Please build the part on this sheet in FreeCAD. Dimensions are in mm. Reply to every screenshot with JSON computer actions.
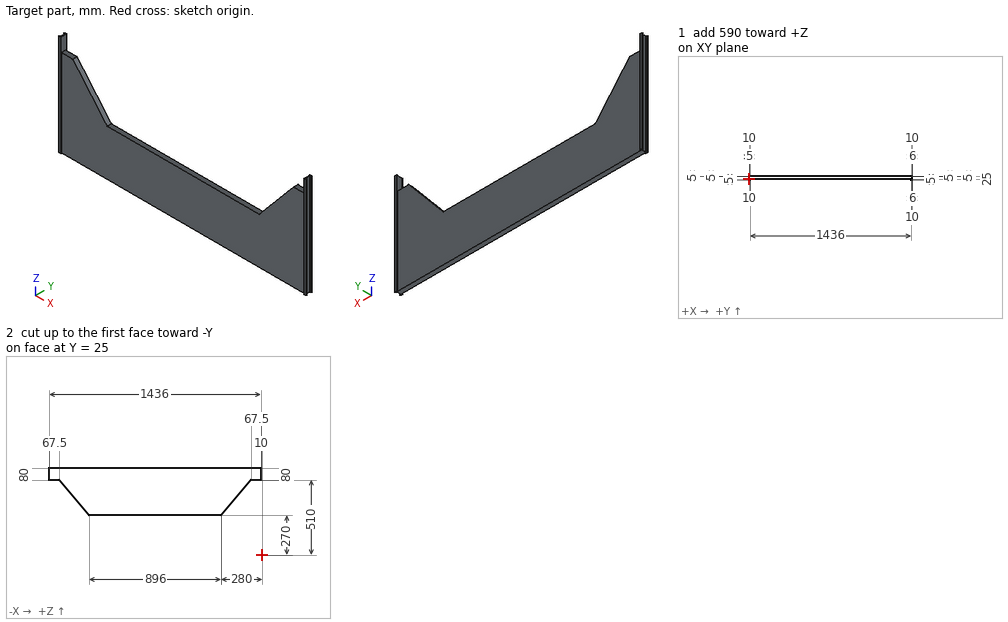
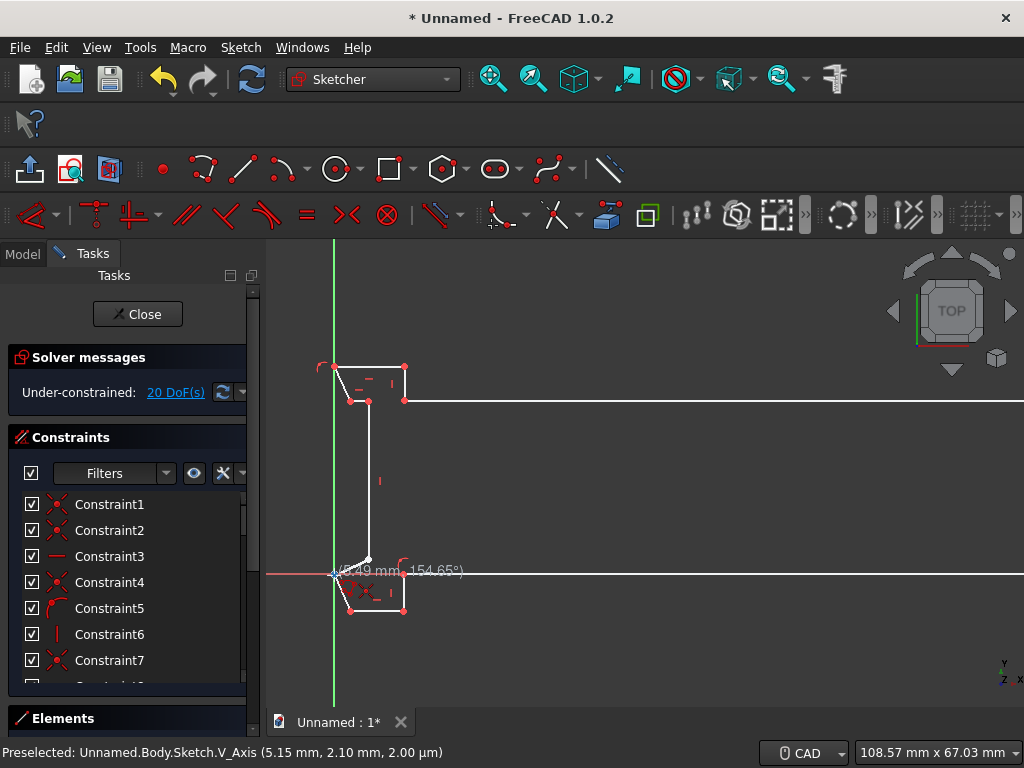
{"action": "left_click", "coordinate": [334, 574]}
{"action": "key", "text": "Escape"}
{"action": "key", "text": "Escape"}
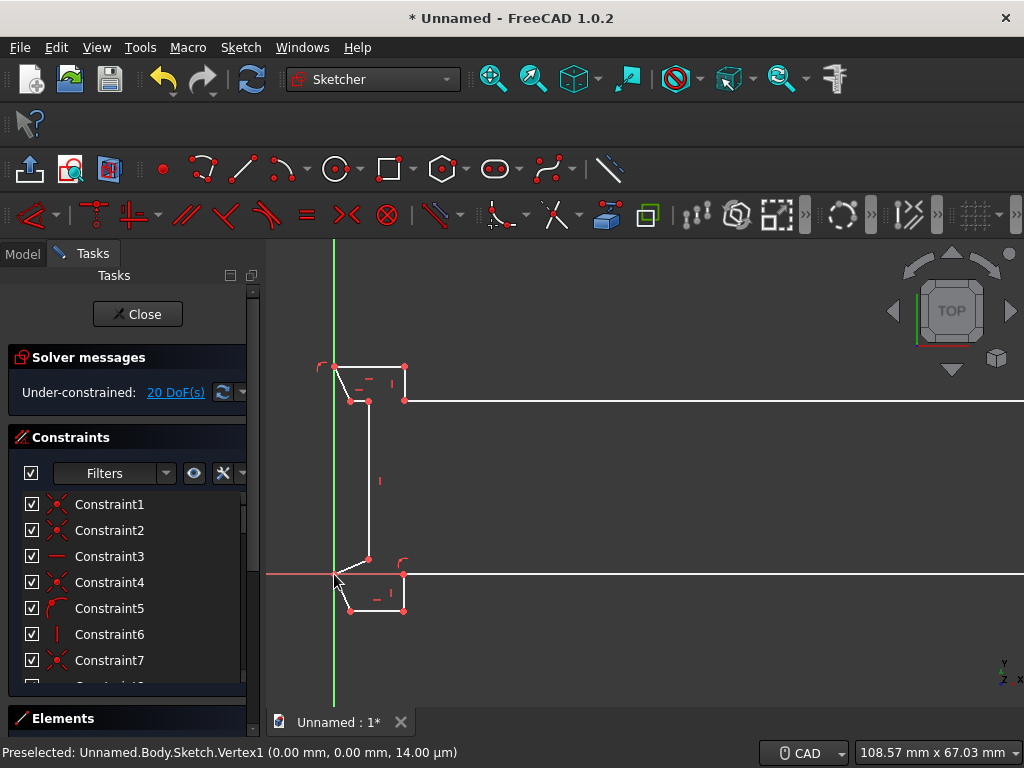
{"action": "left_click", "coordinate": [346, 600]}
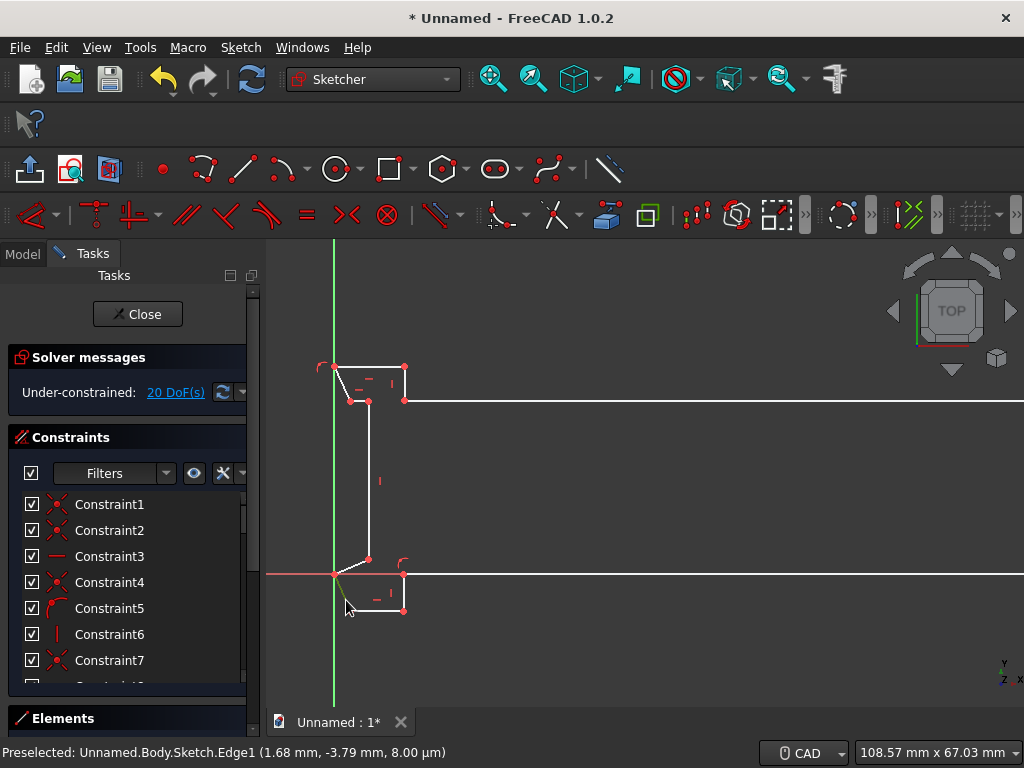
{"action": "key", "text": "v"}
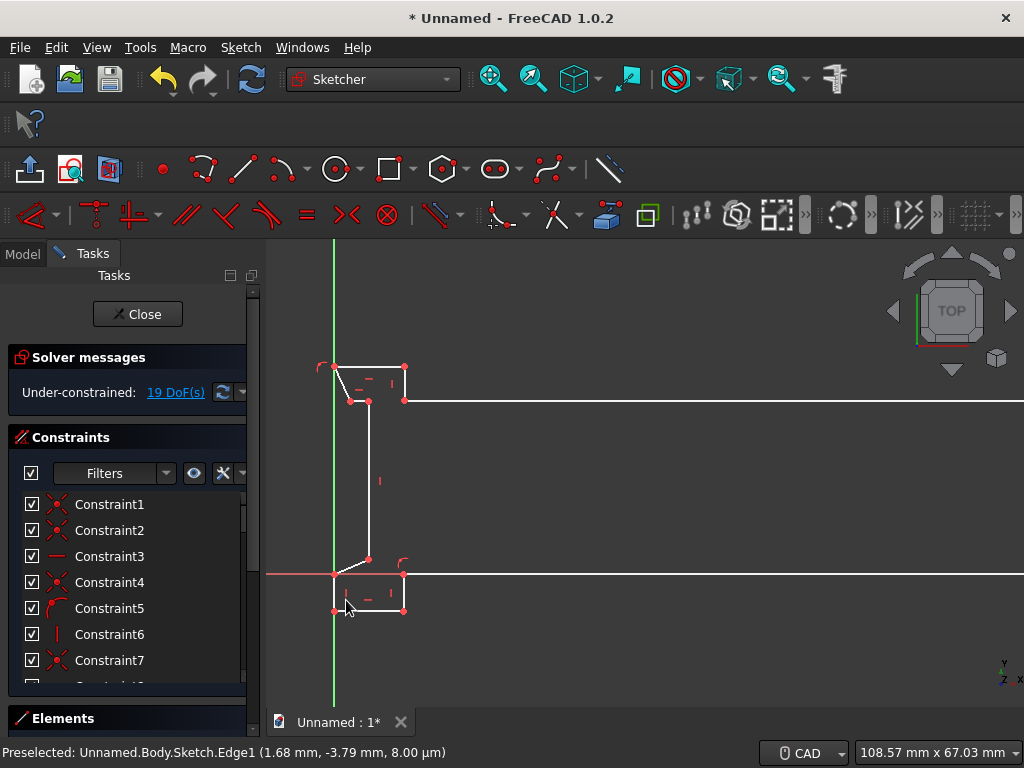
{"action": "scroll", "coordinate": [323, 472], "scroll_direction": "down", "scroll_amount": 15}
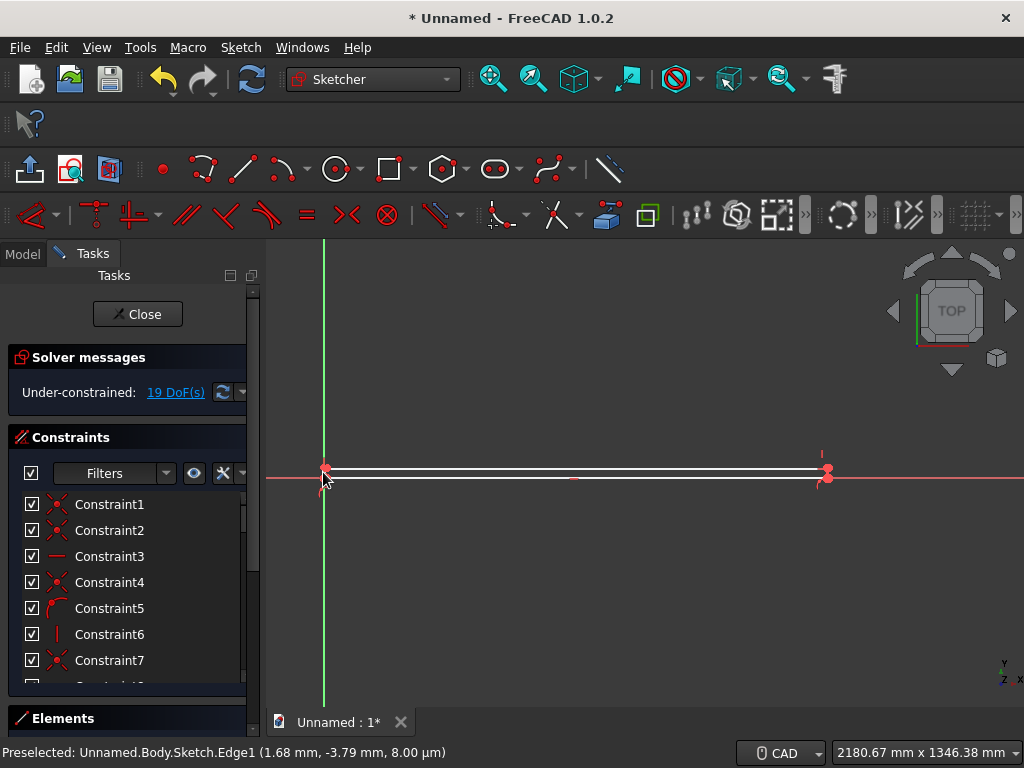
{"action": "scroll", "coordinate": [828, 477], "scroll_direction": "up", "scroll_amount": 13}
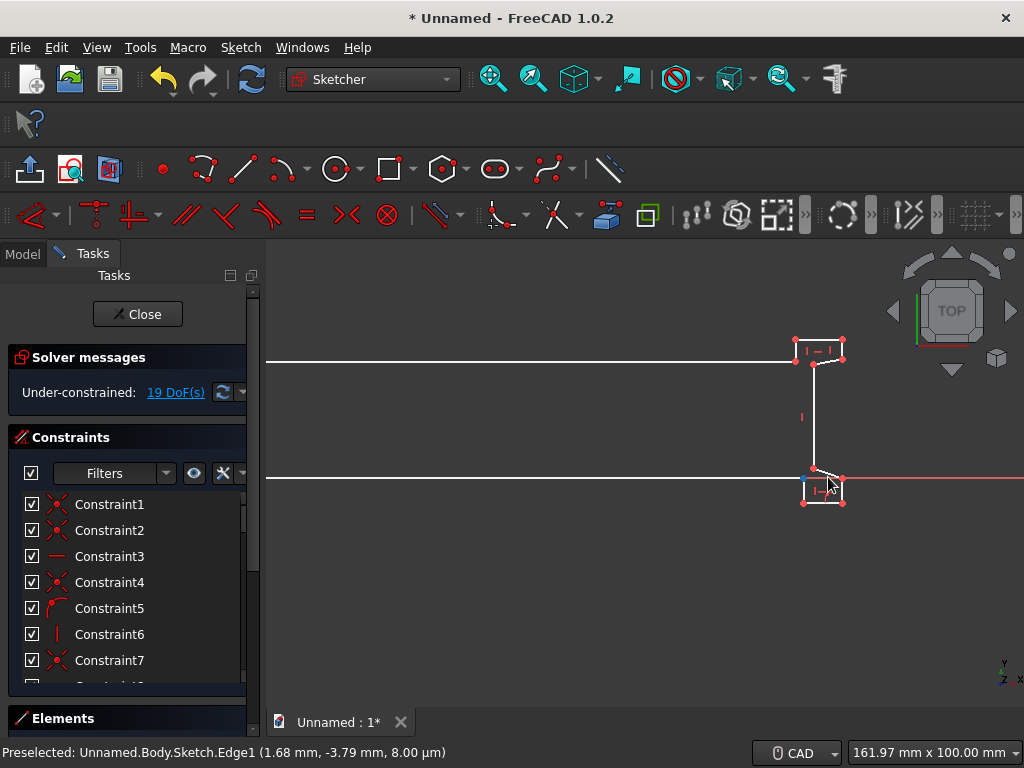
{"action": "left_click", "coordinate": [822, 472]}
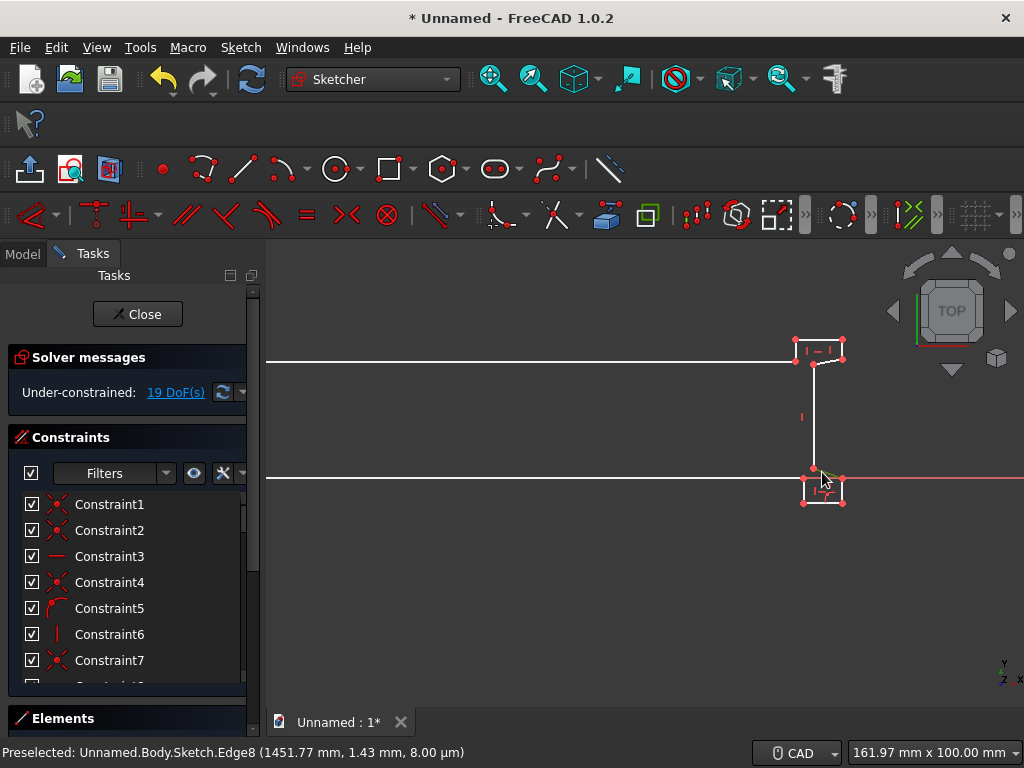
{"action": "left_click", "coordinate": [160, 216]}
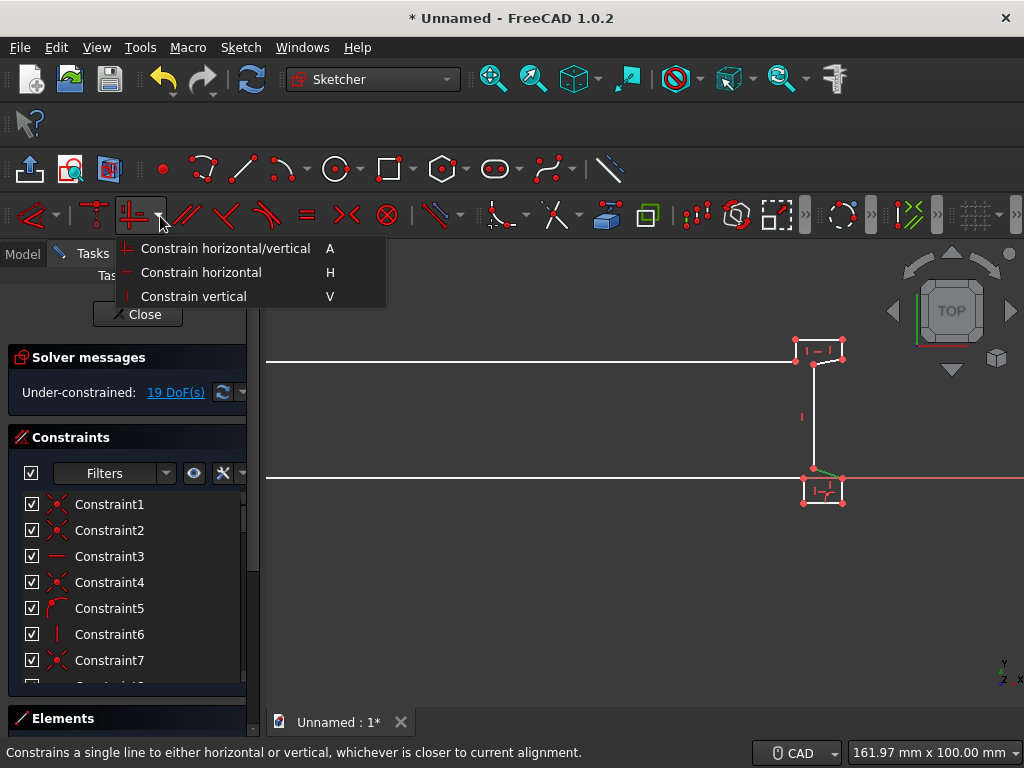
{"action": "left_click", "coordinate": [251, 272]}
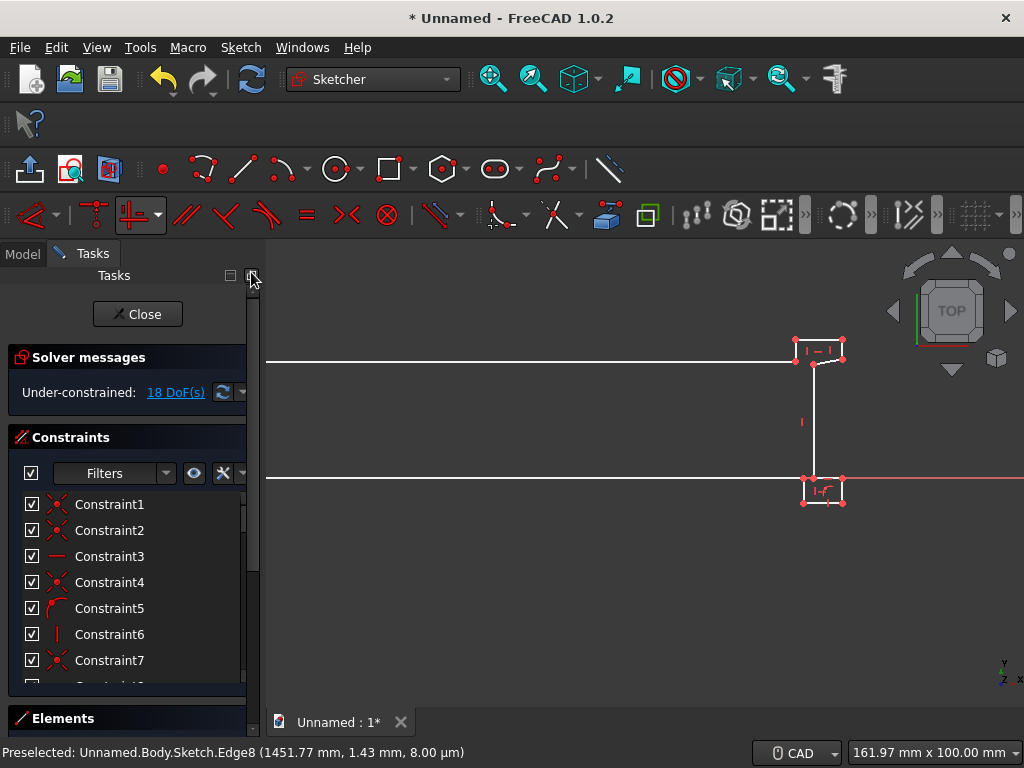
{"action": "left_click", "coordinate": [825, 362]}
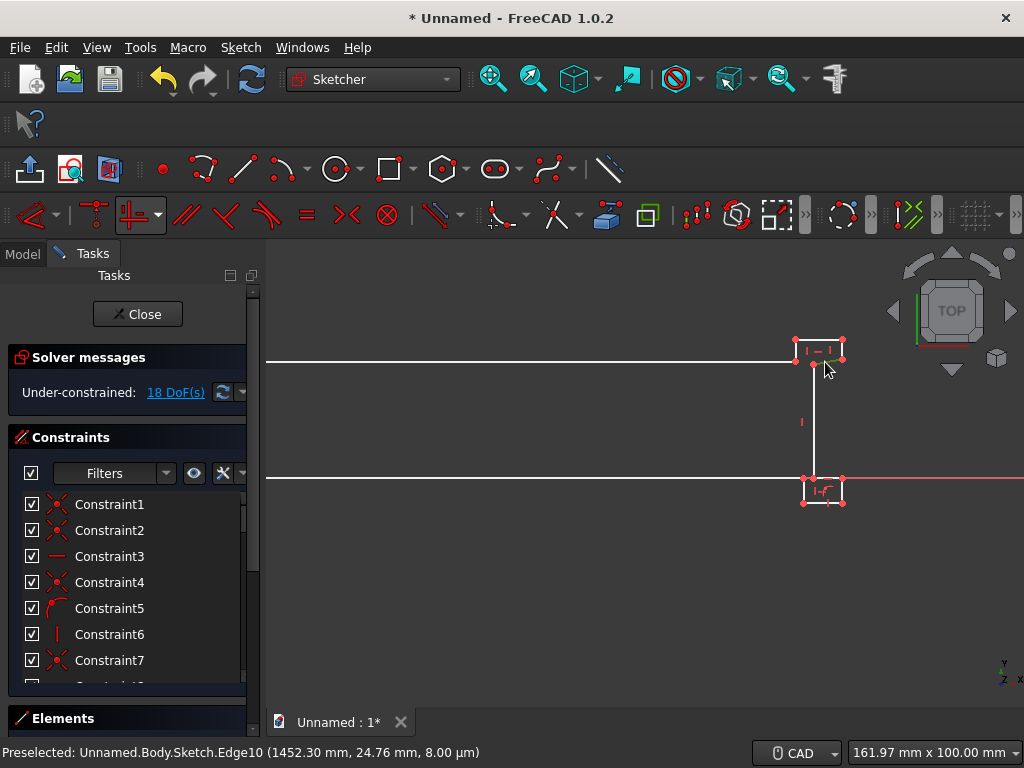
{"action": "key", "text": "h"}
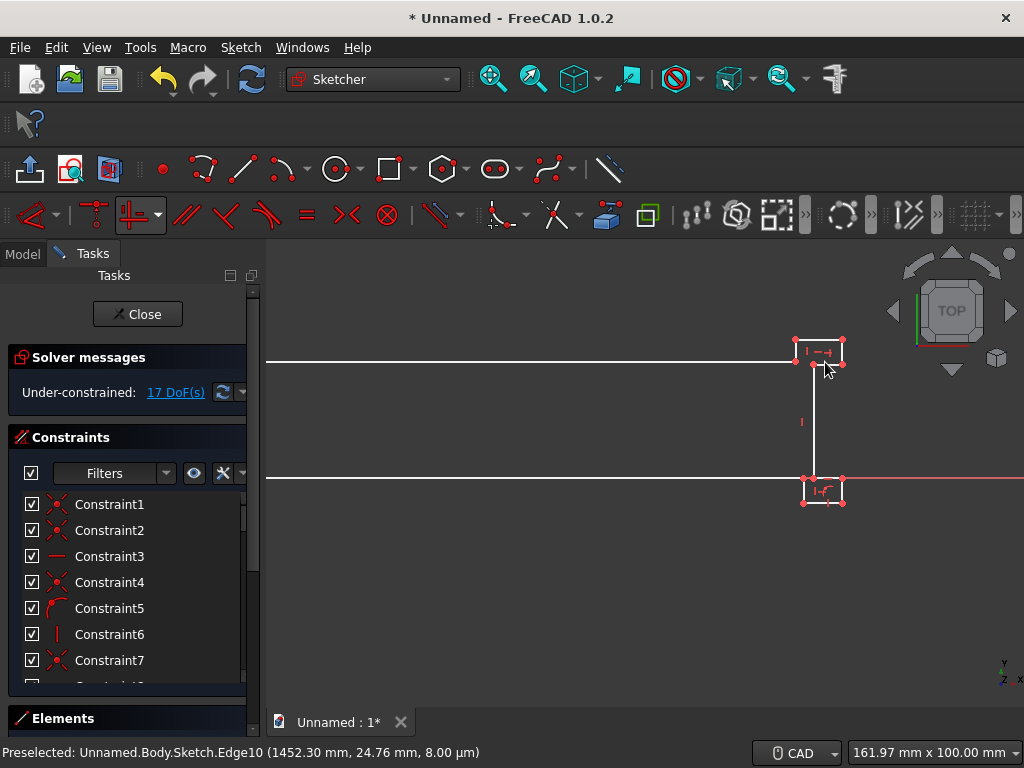
{"action": "scroll", "coordinate": [780, 476], "scroll_direction": "down", "scroll_amount": 14}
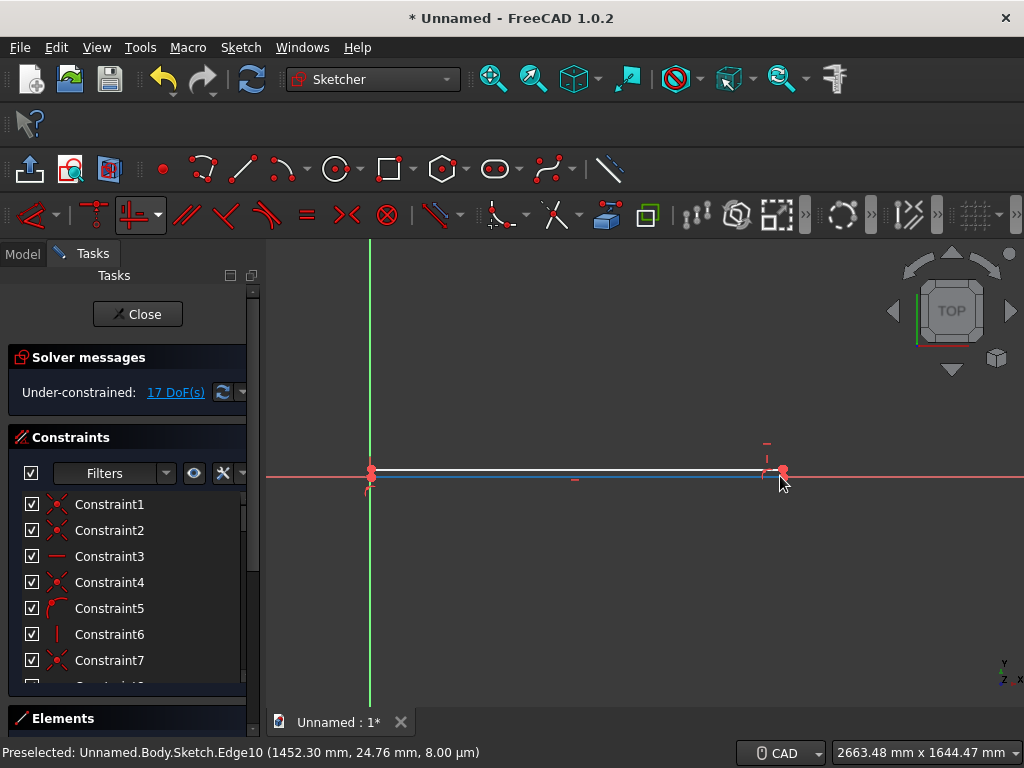
{"action": "scroll", "coordinate": [371, 469], "scroll_direction": "up", "scroll_amount": 14}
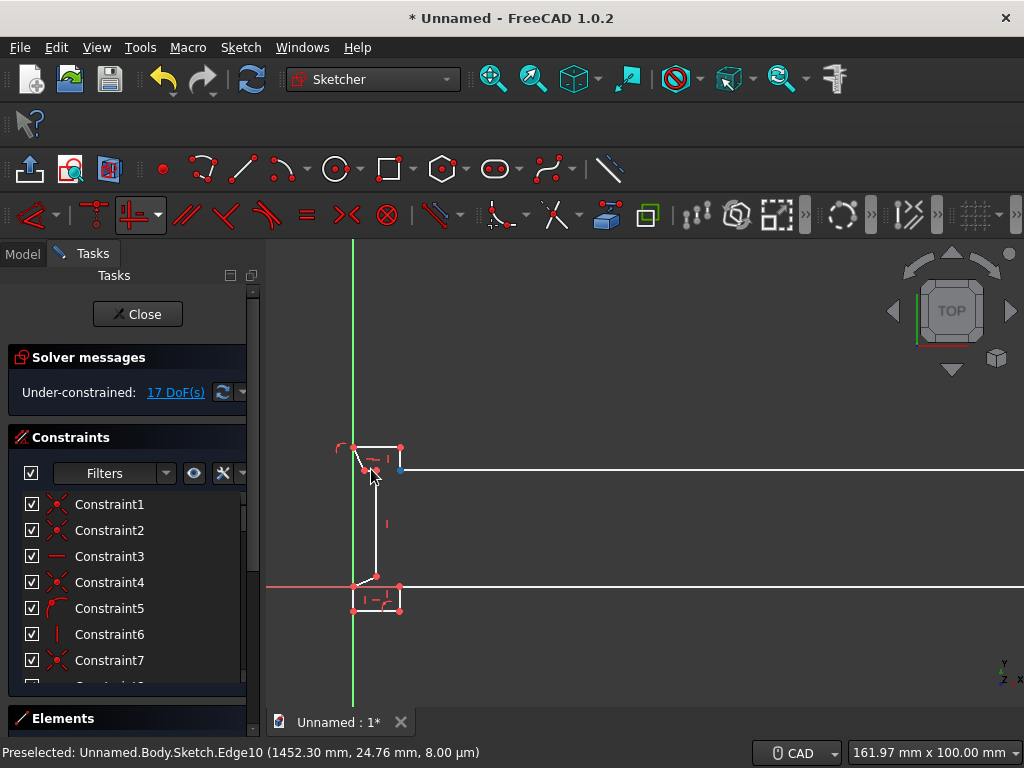
{"action": "left_click", "coordinate": [361, 464]}